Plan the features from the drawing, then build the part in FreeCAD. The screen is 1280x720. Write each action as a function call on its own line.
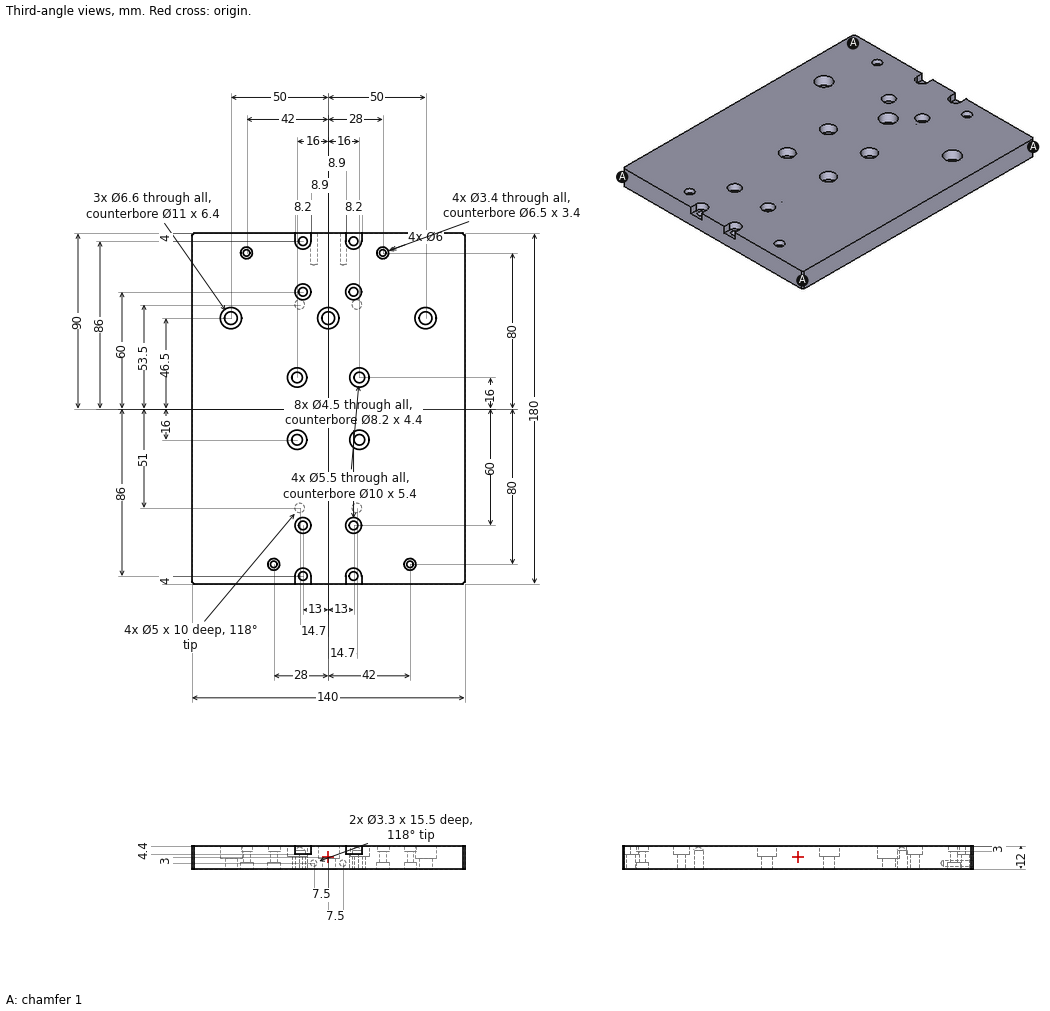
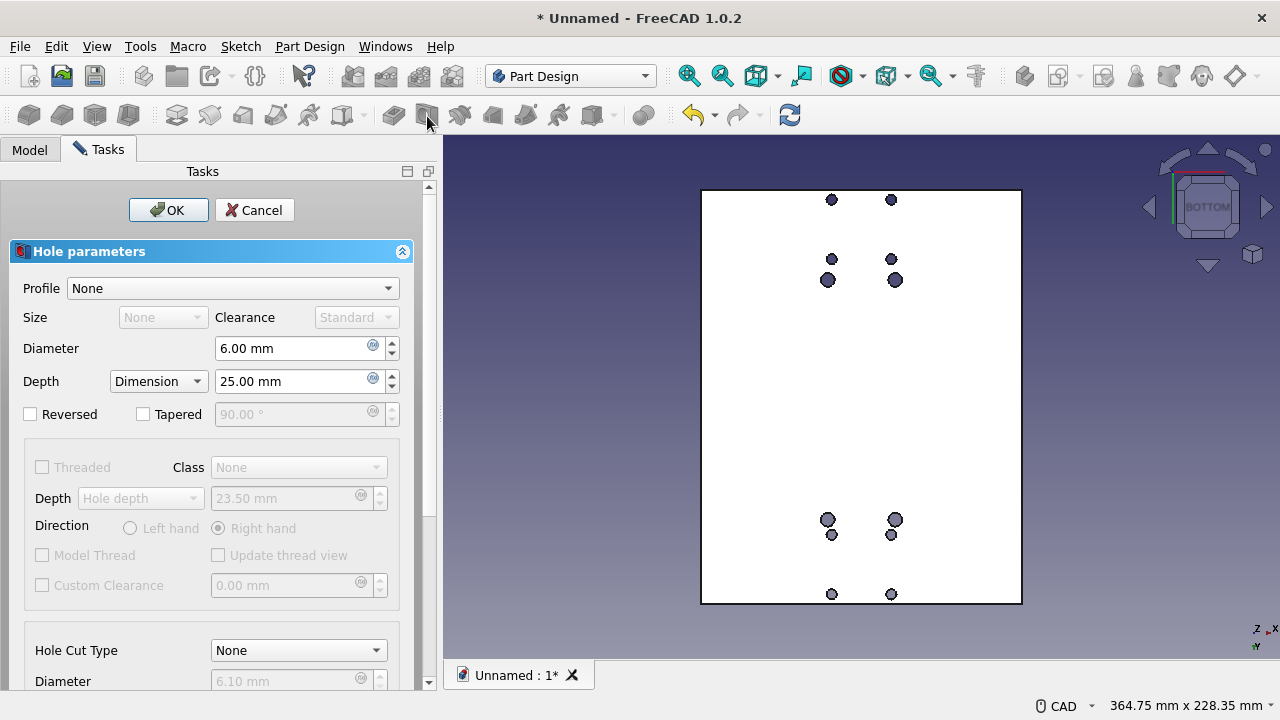
triple_click(300, 348)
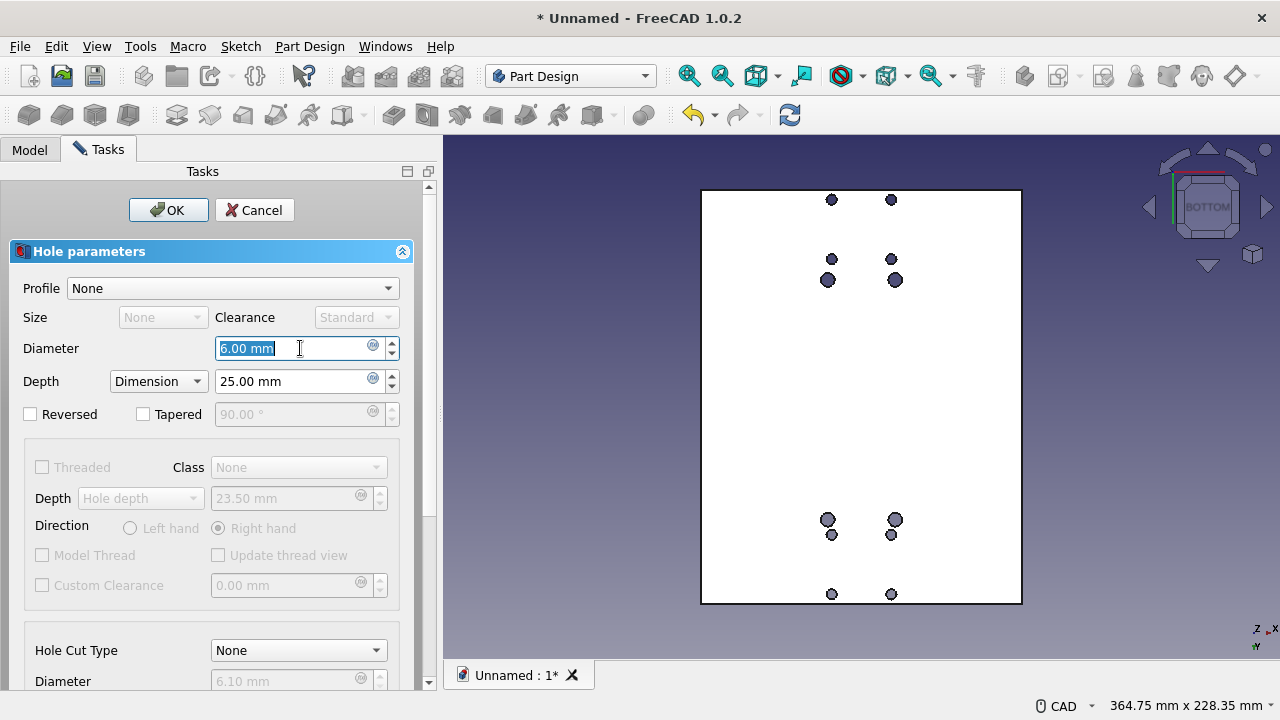
text(5)
key(Tab)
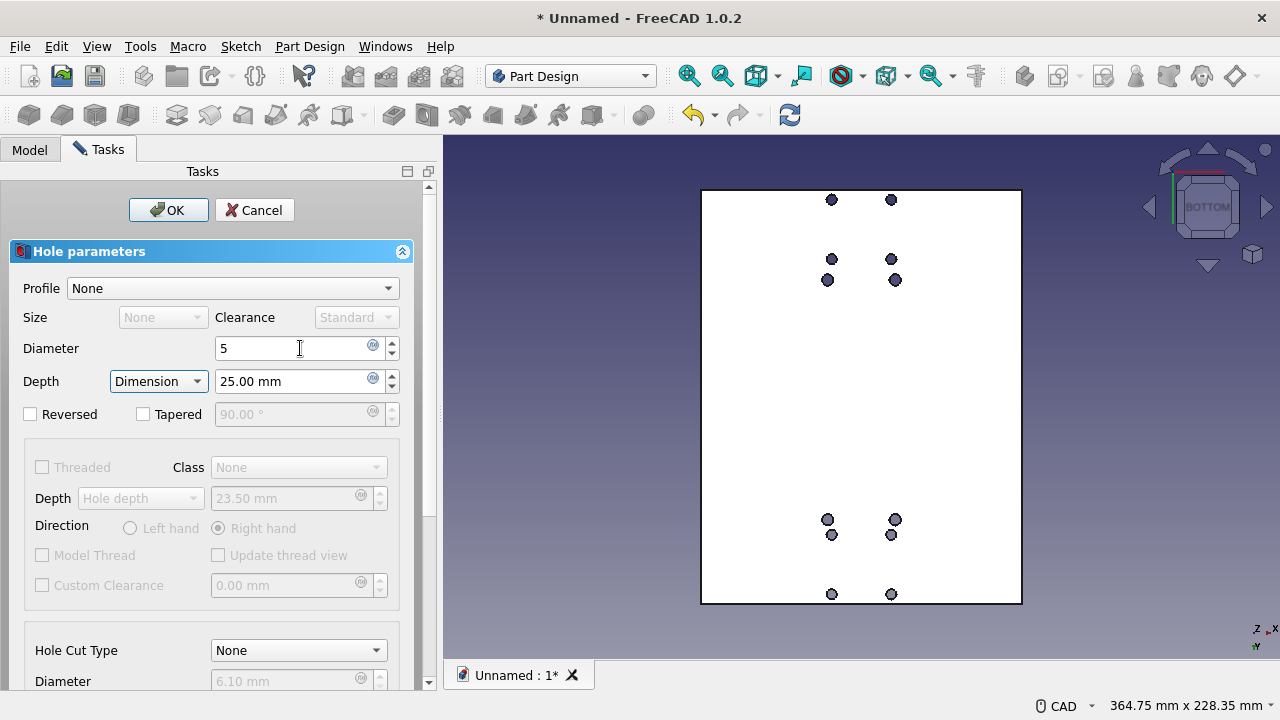
triple_click(300, 382)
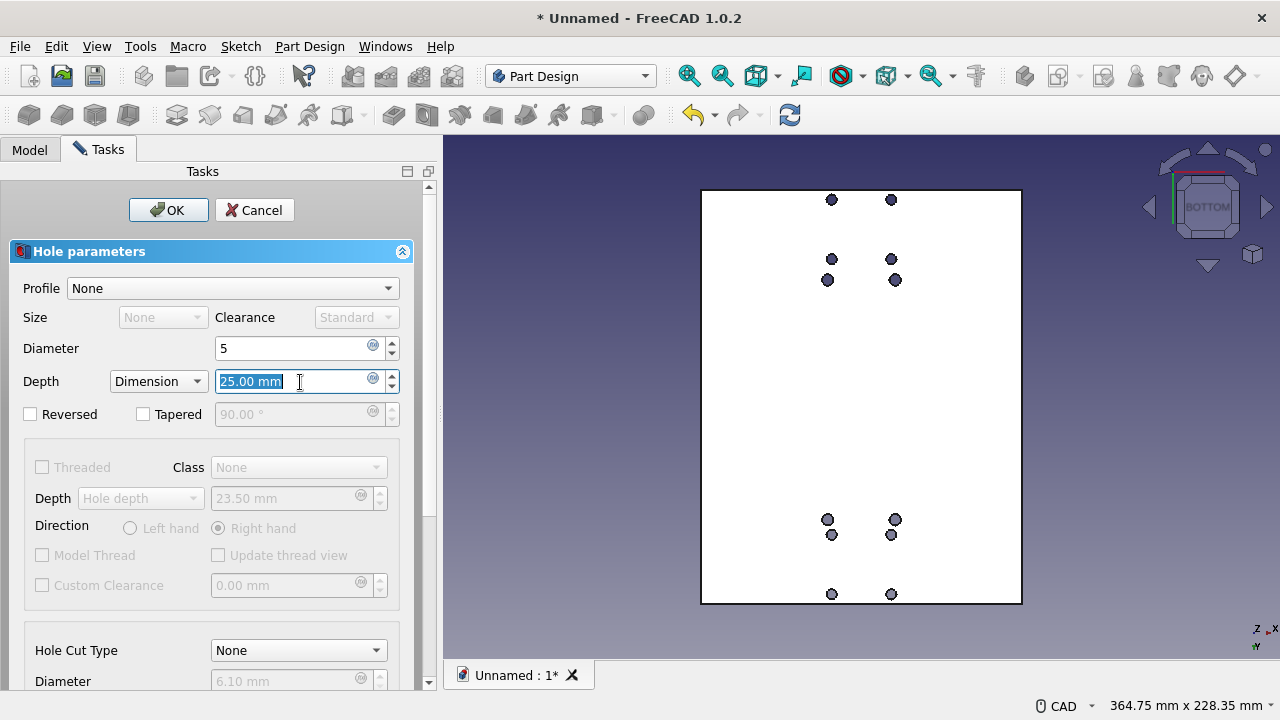
text(10)
key(Tab)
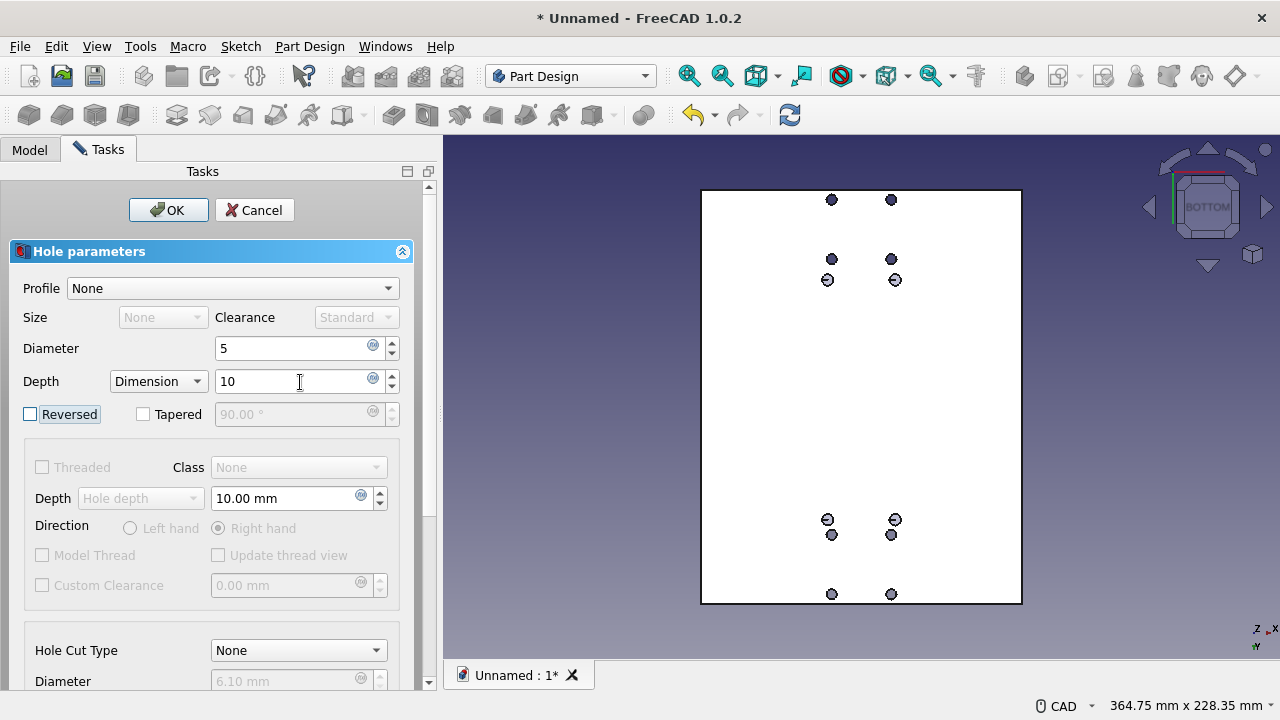
click(169, 210)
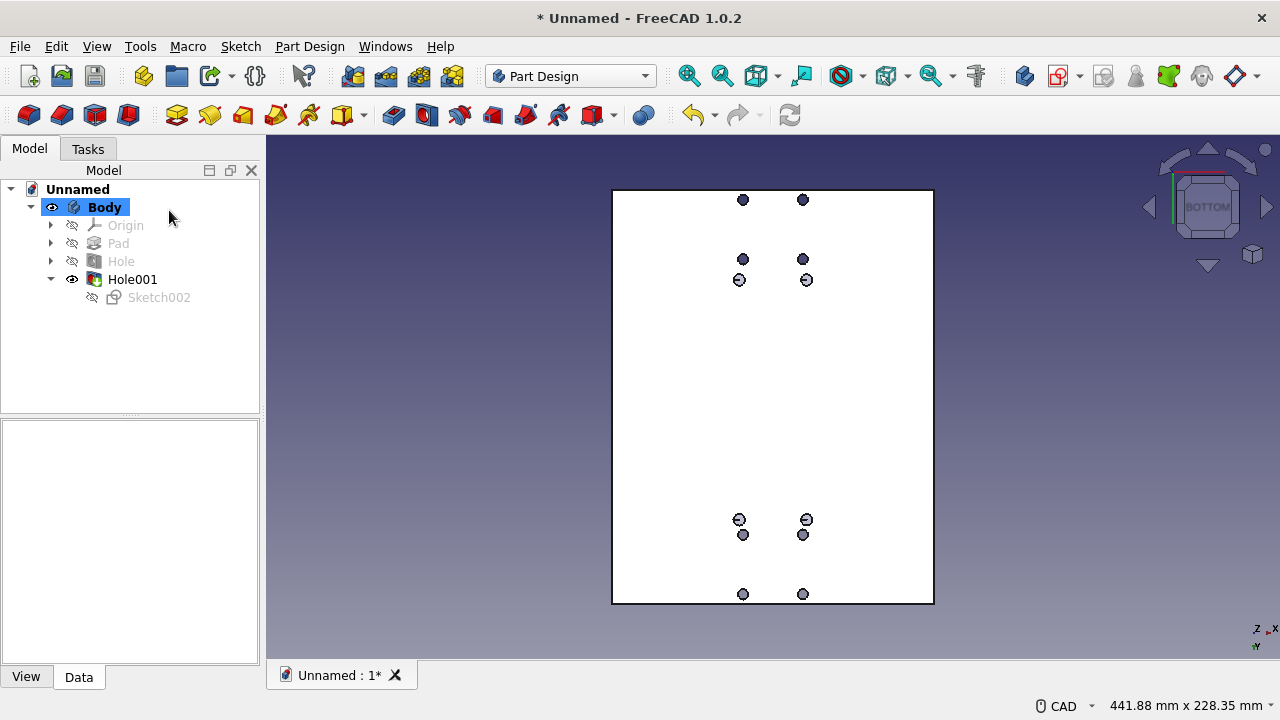
key(0)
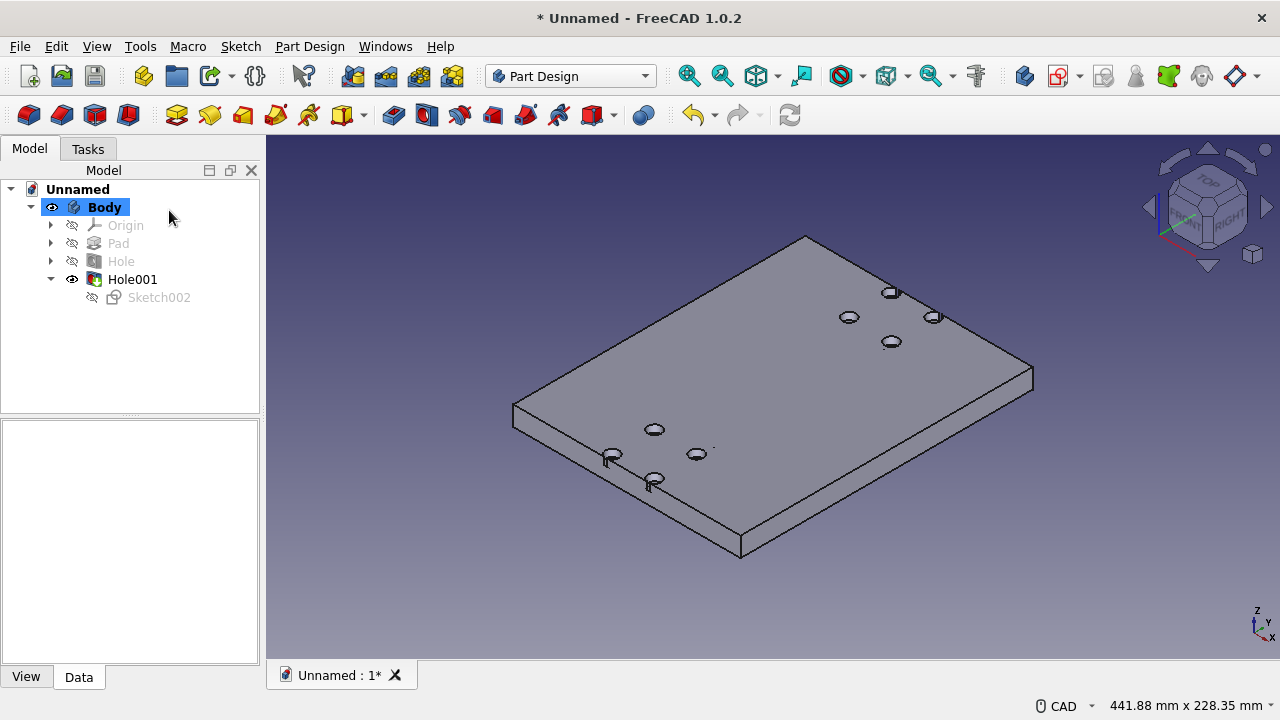
click(773, 385)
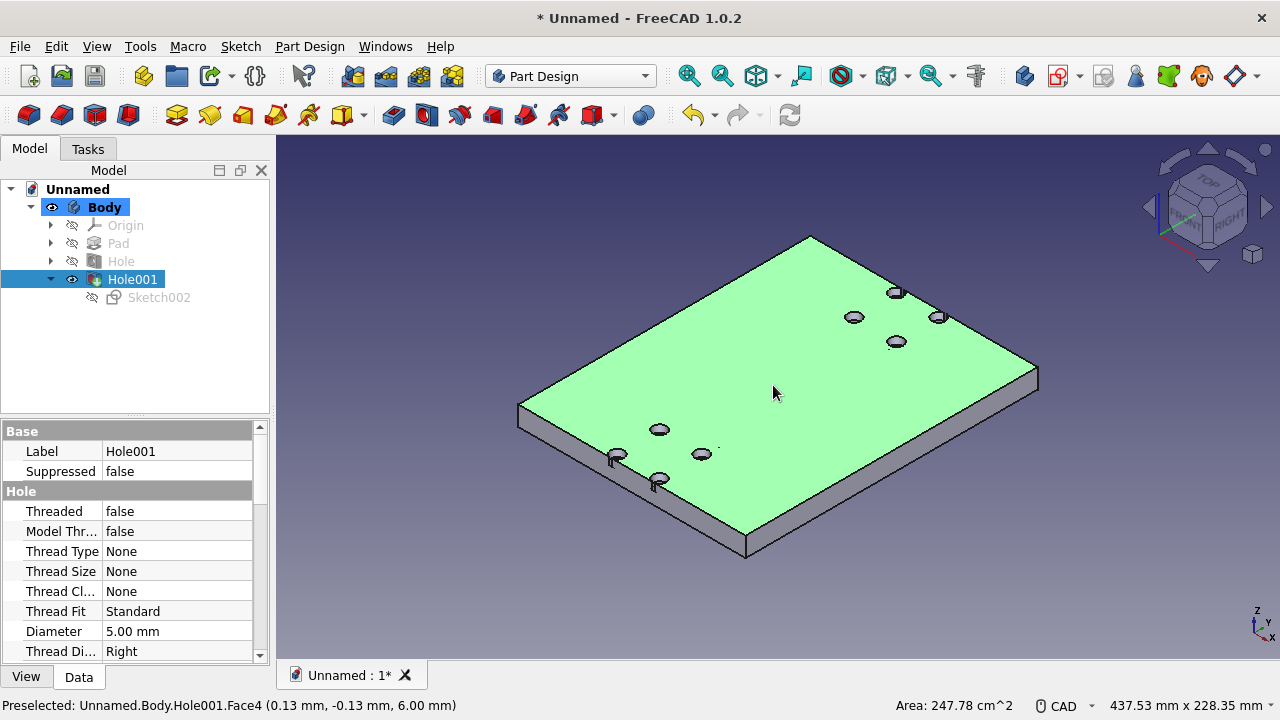
click(1058, 76)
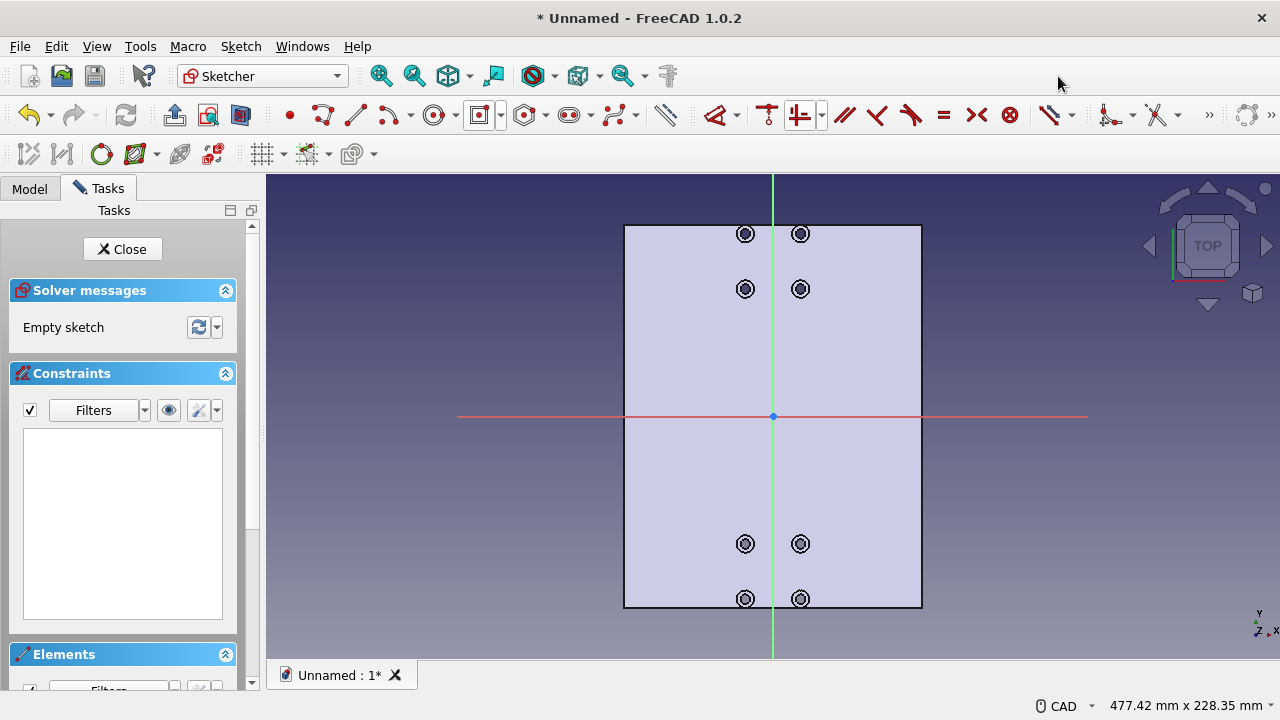
scroll(795, 416, up, 7)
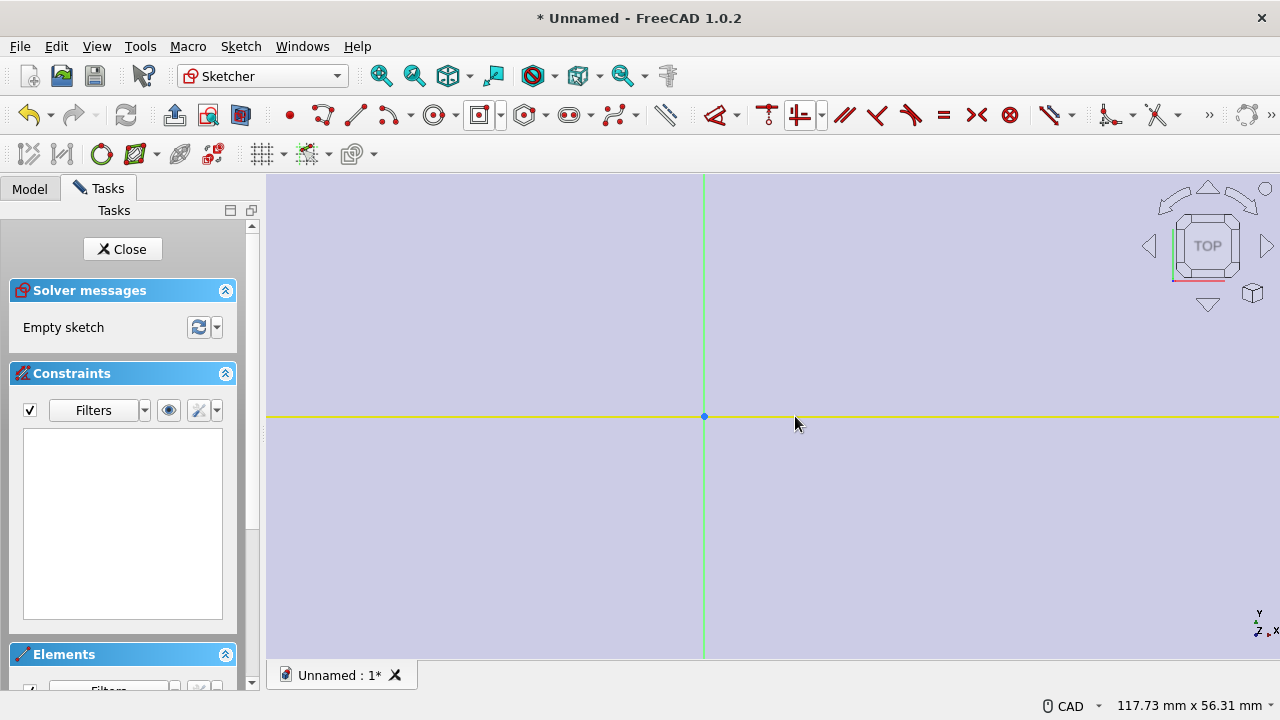
click(434, 116)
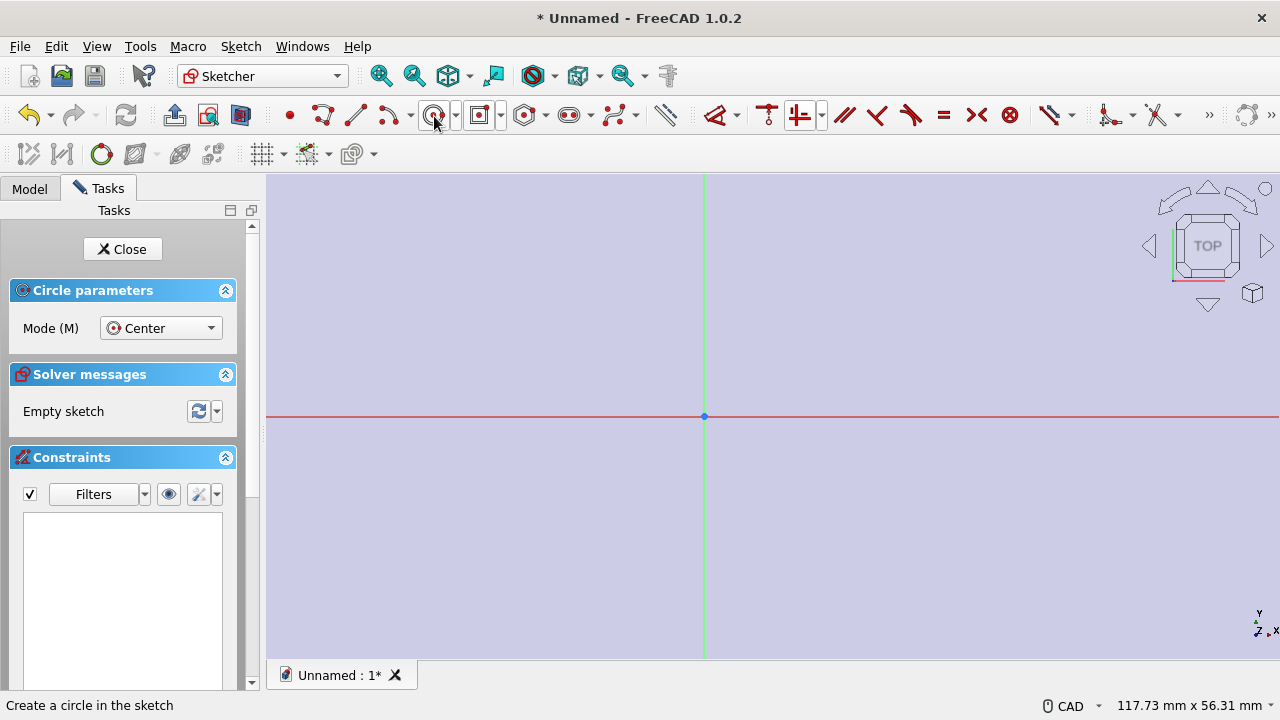
click(842, 279)
click(859, 262)